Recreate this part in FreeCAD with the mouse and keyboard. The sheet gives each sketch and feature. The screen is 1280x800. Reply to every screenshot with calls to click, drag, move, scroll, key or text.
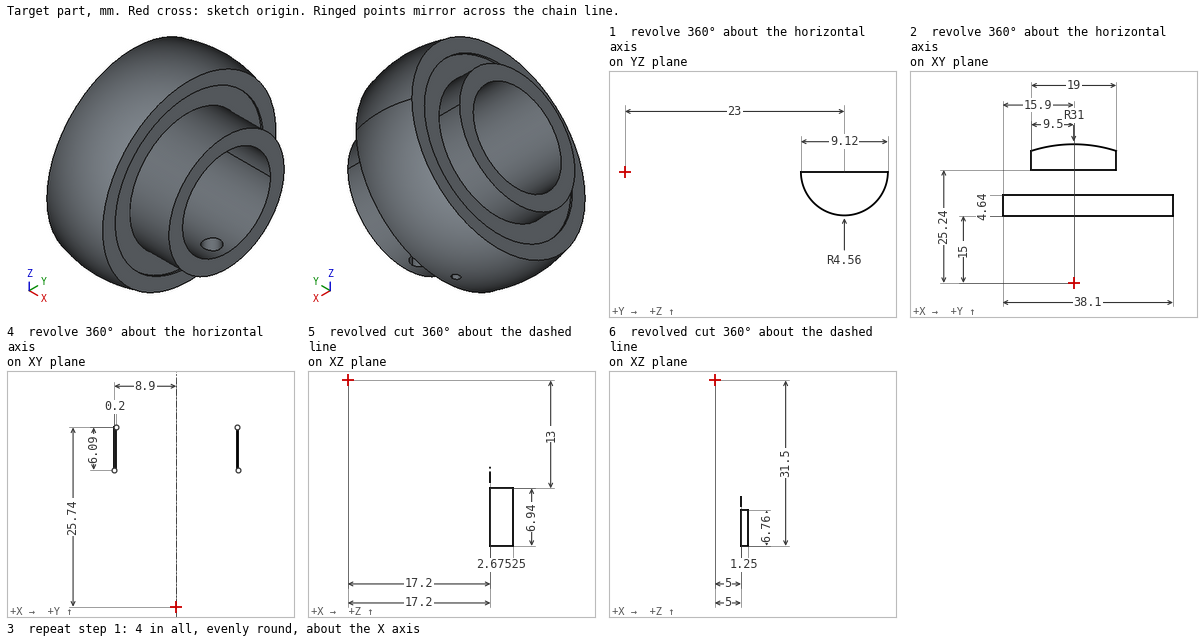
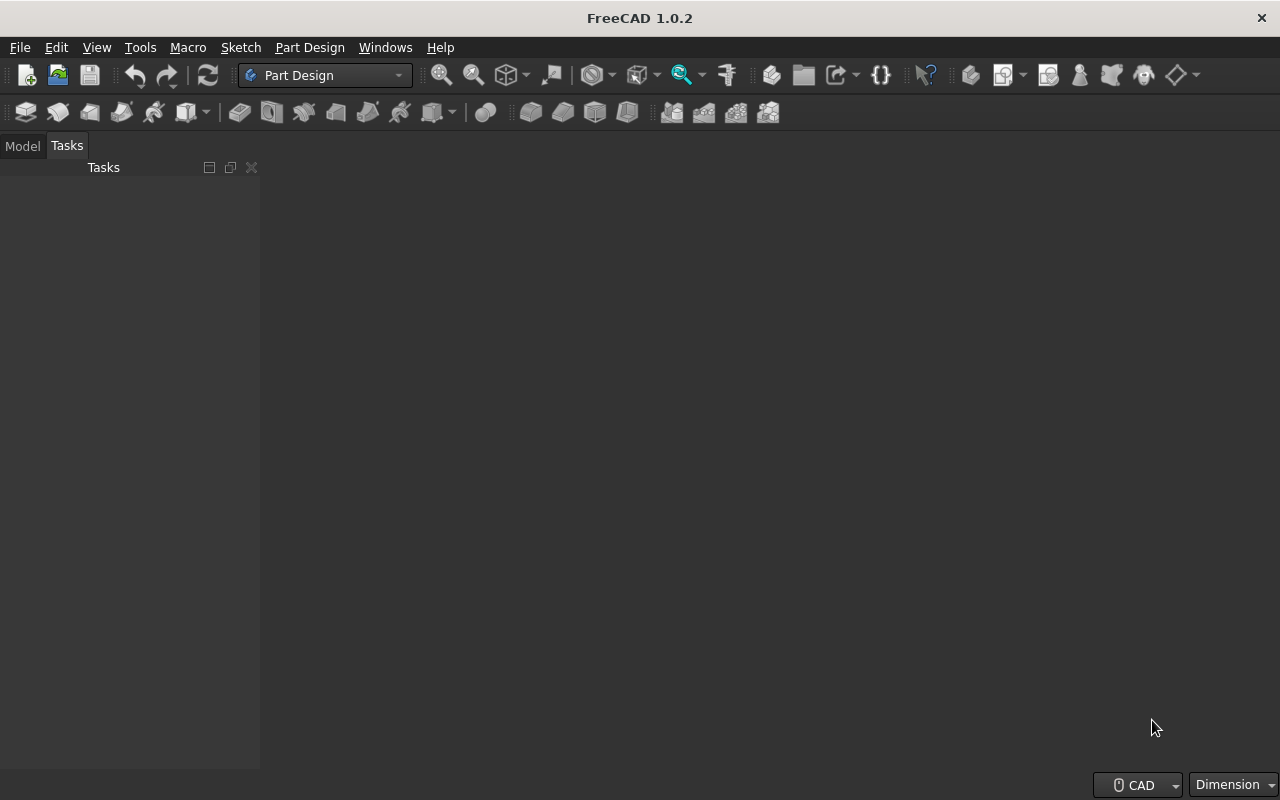
click(26, 76)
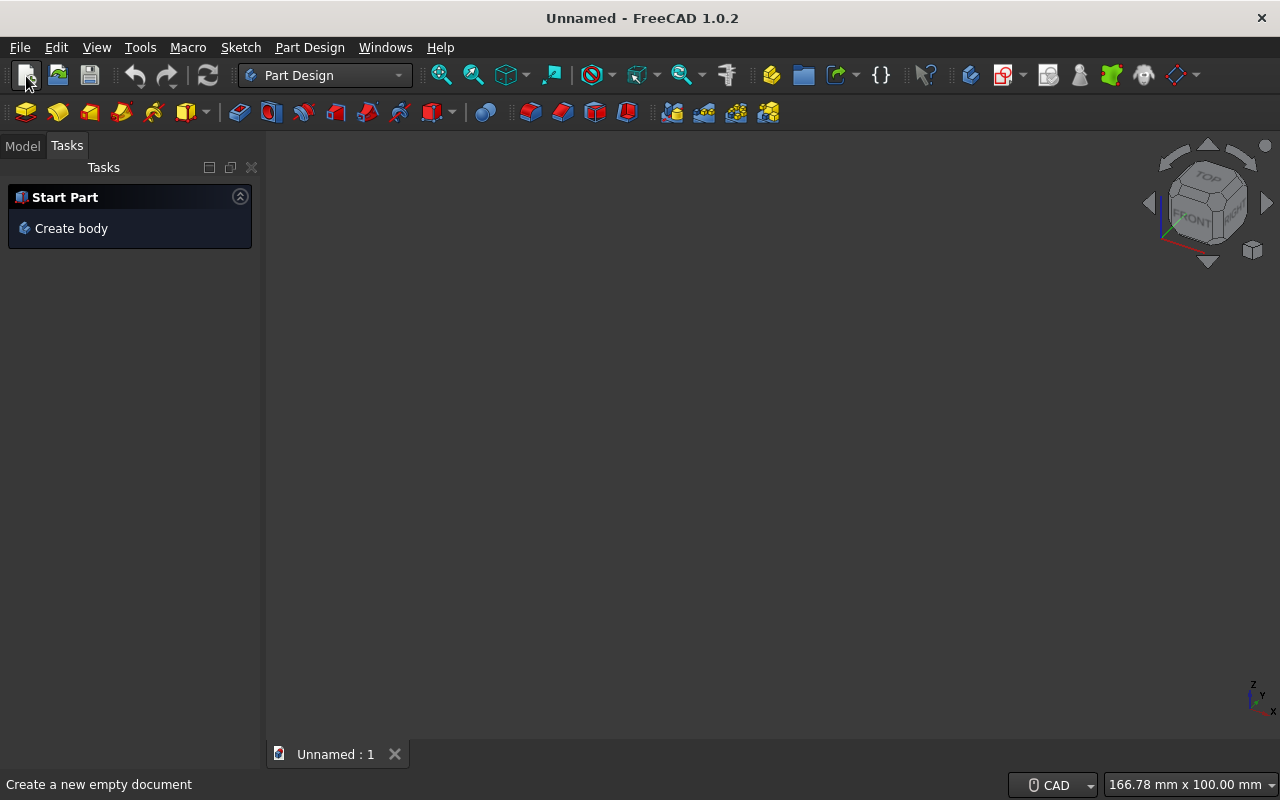
click(1004, 76)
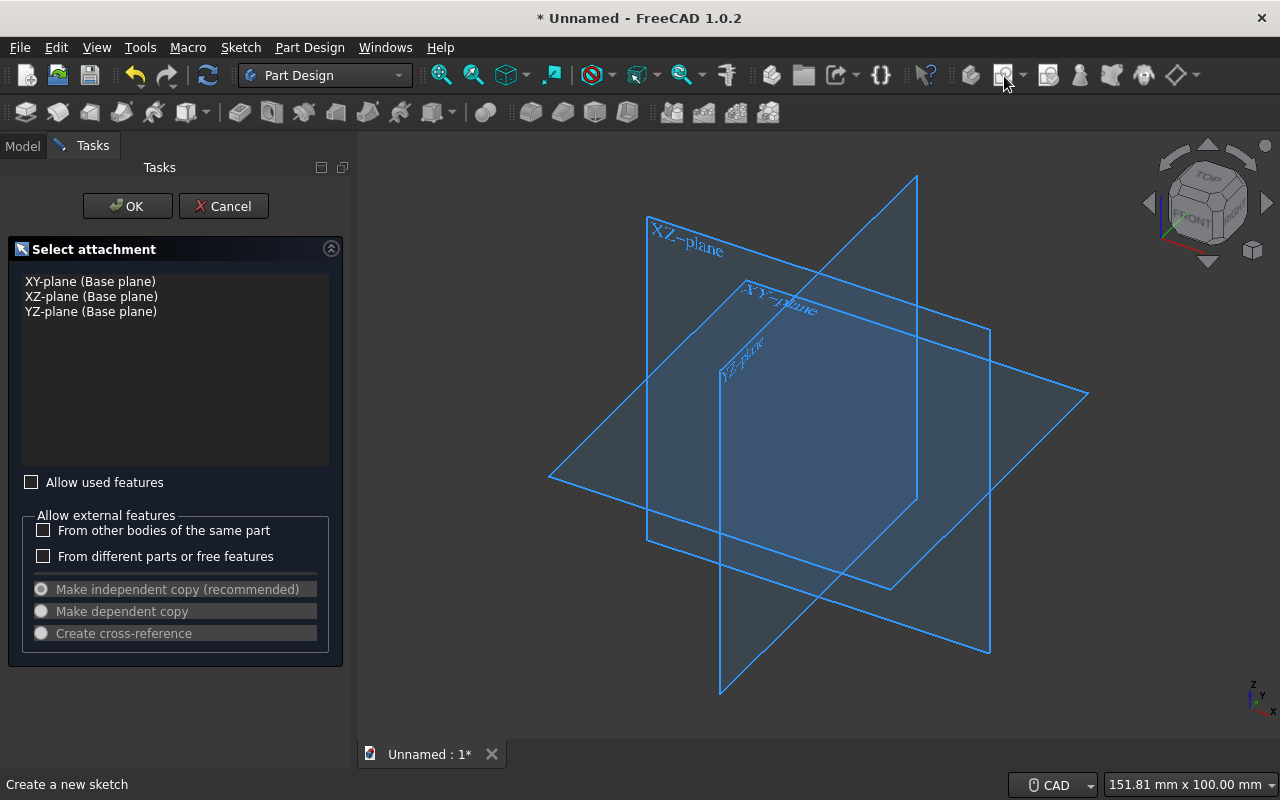
click(82, 312)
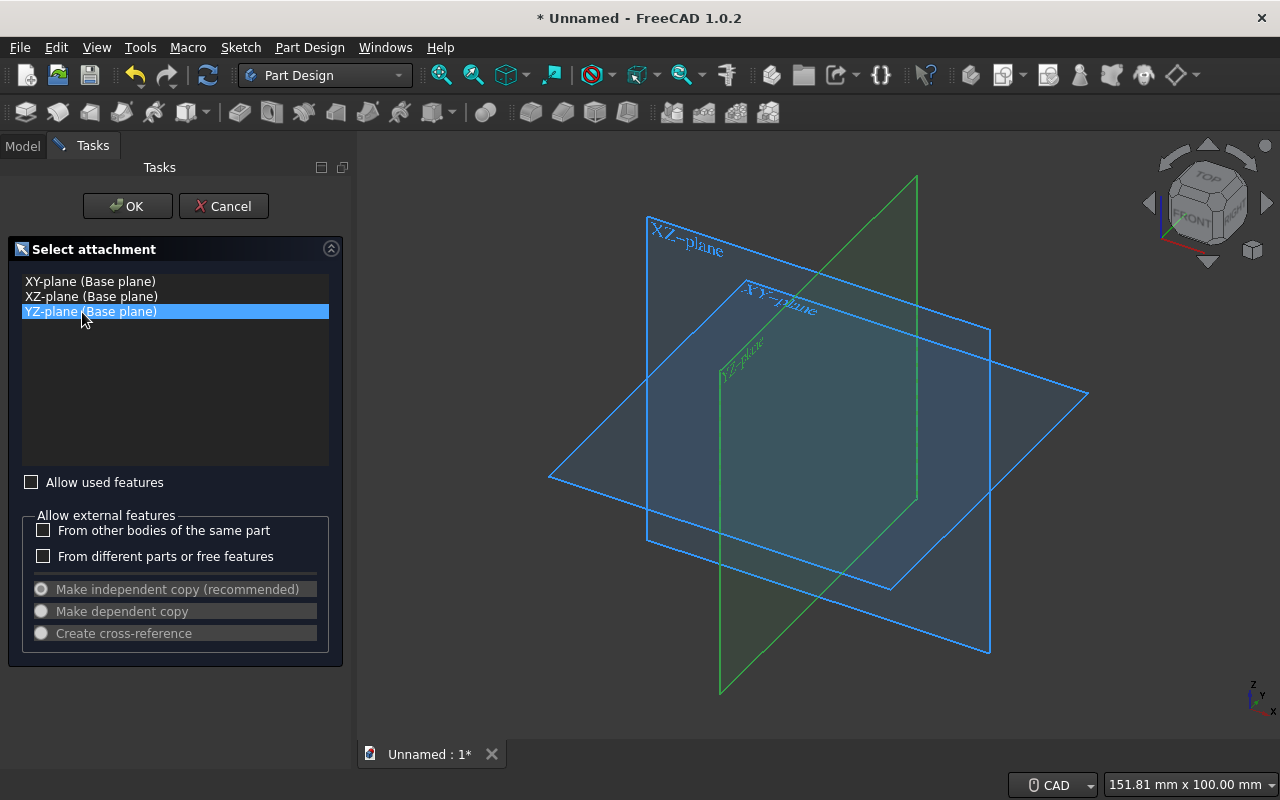
click(128, 206)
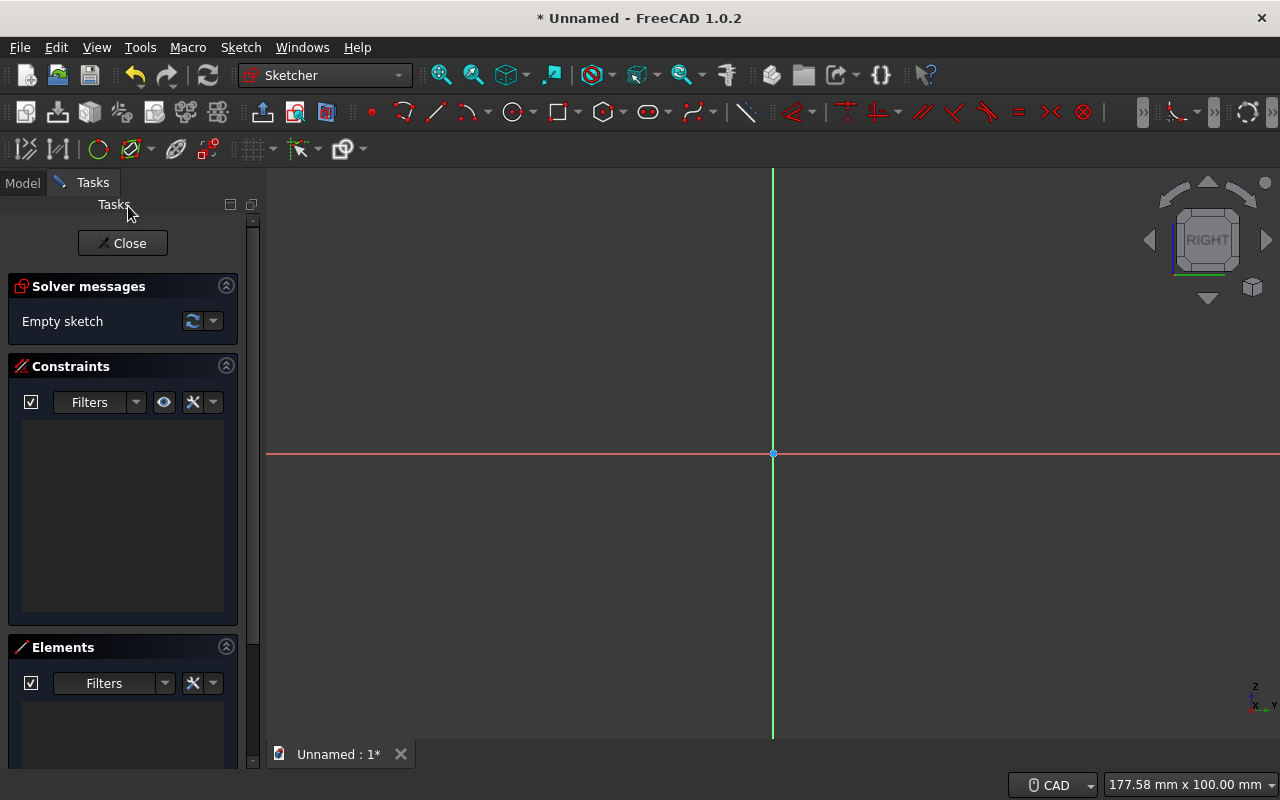
scroll(924, 468, up, 12)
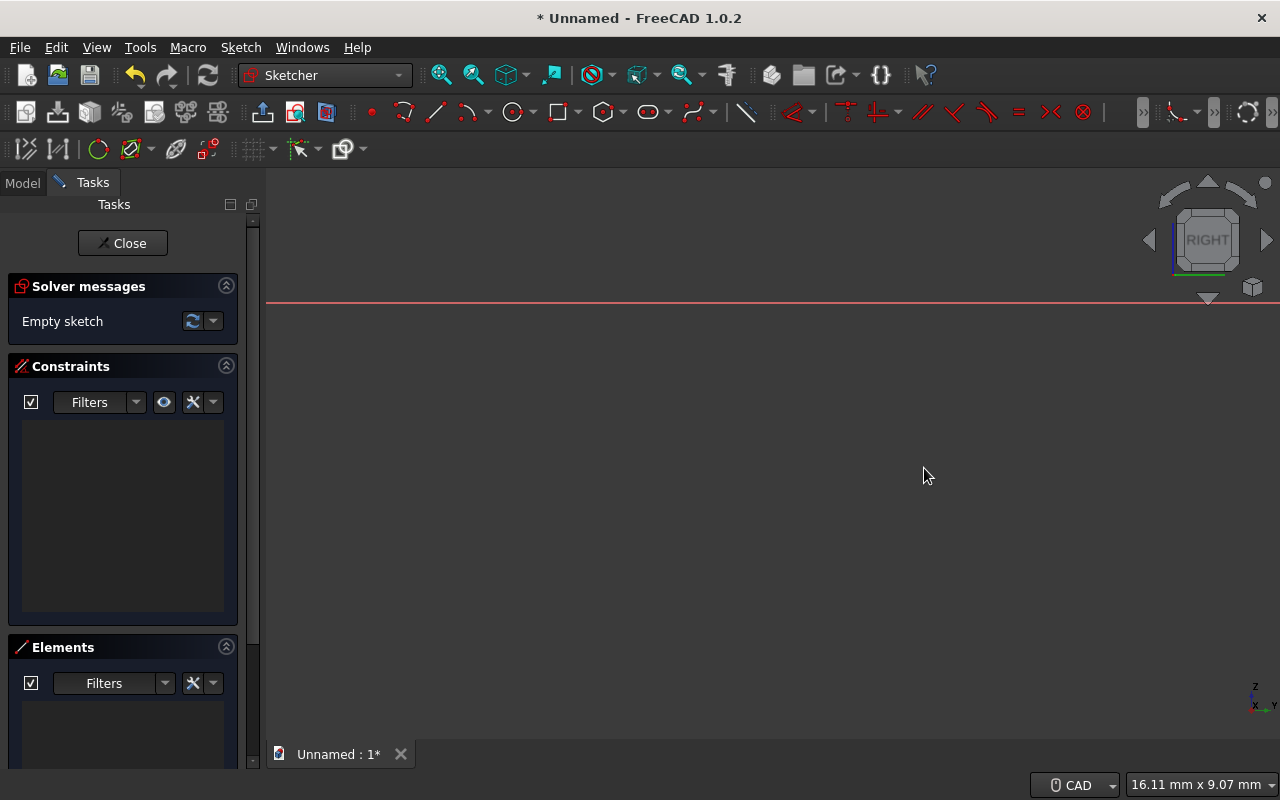
click(436, 112)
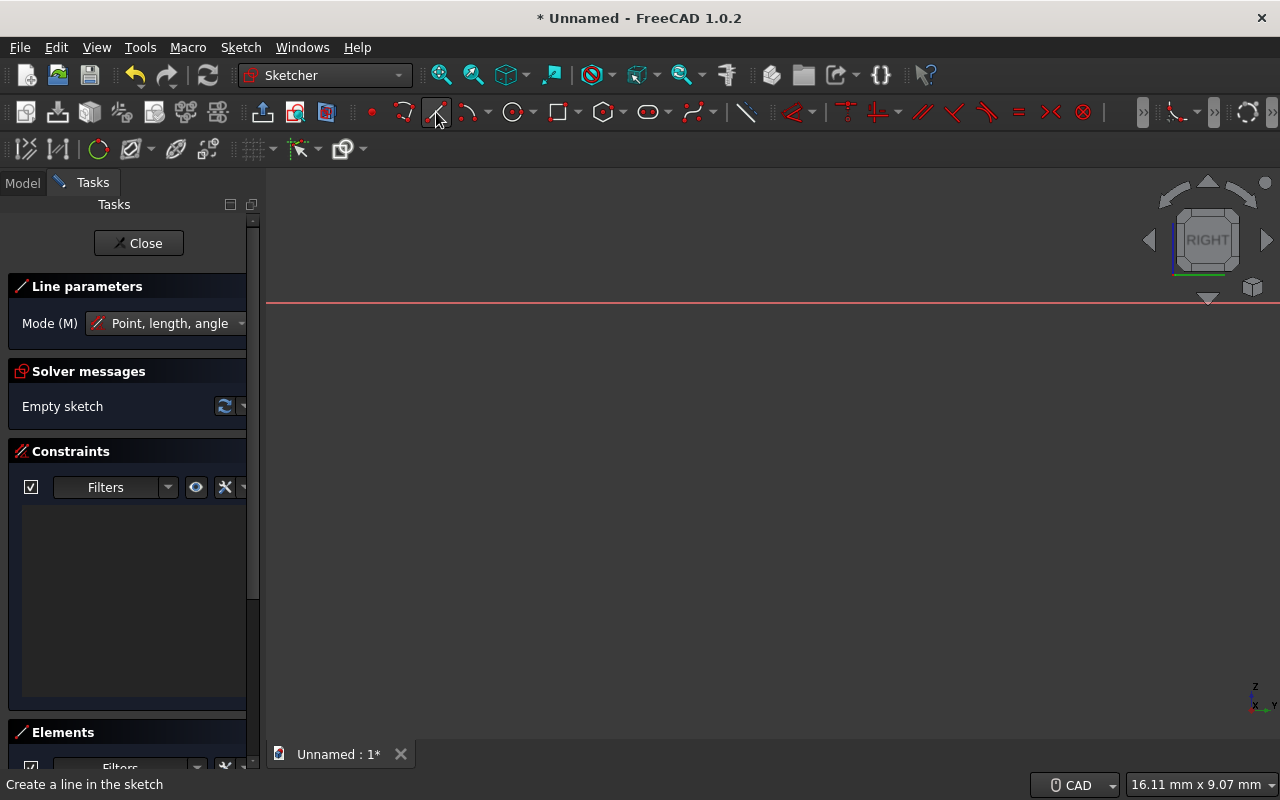
click(988, 303)
click(414, 312)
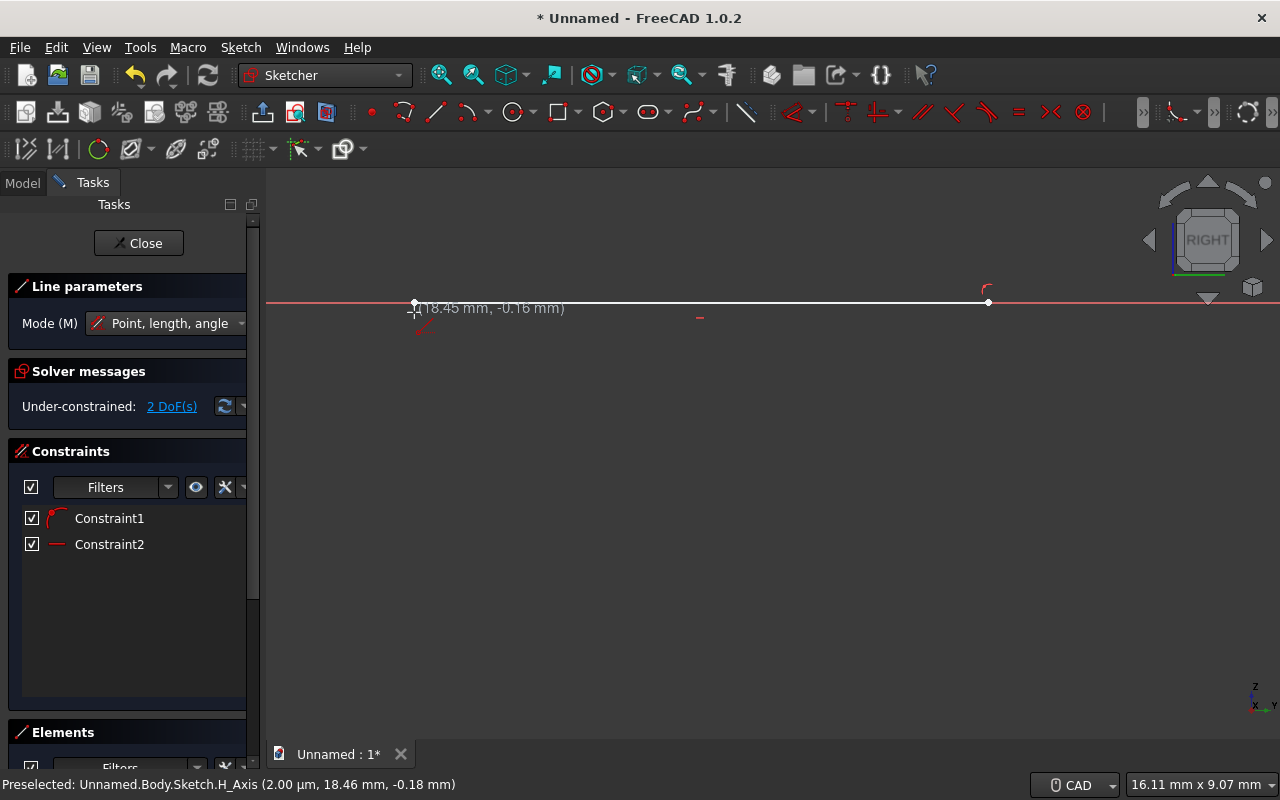
key(g)
key(3)
key(a)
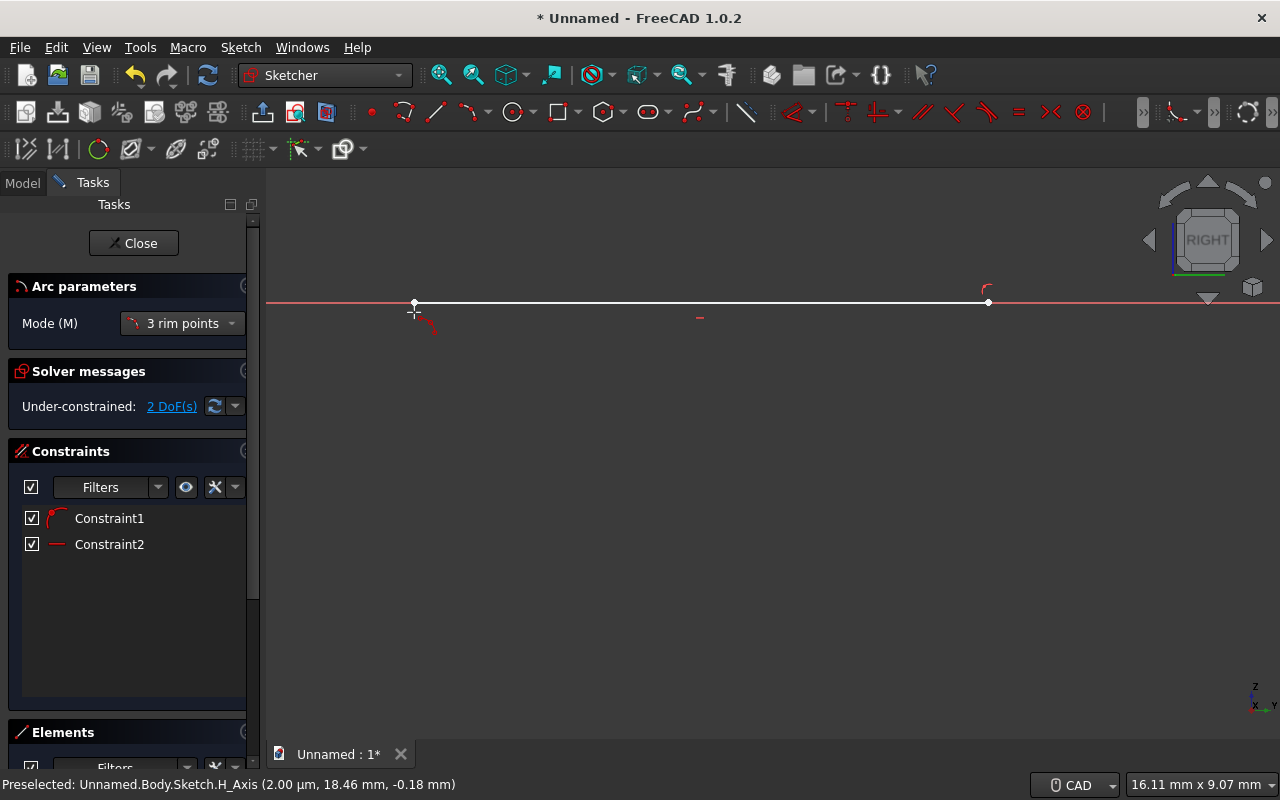
click(414, 312)
click(988, 303)
click(701, 590)
key(Escape)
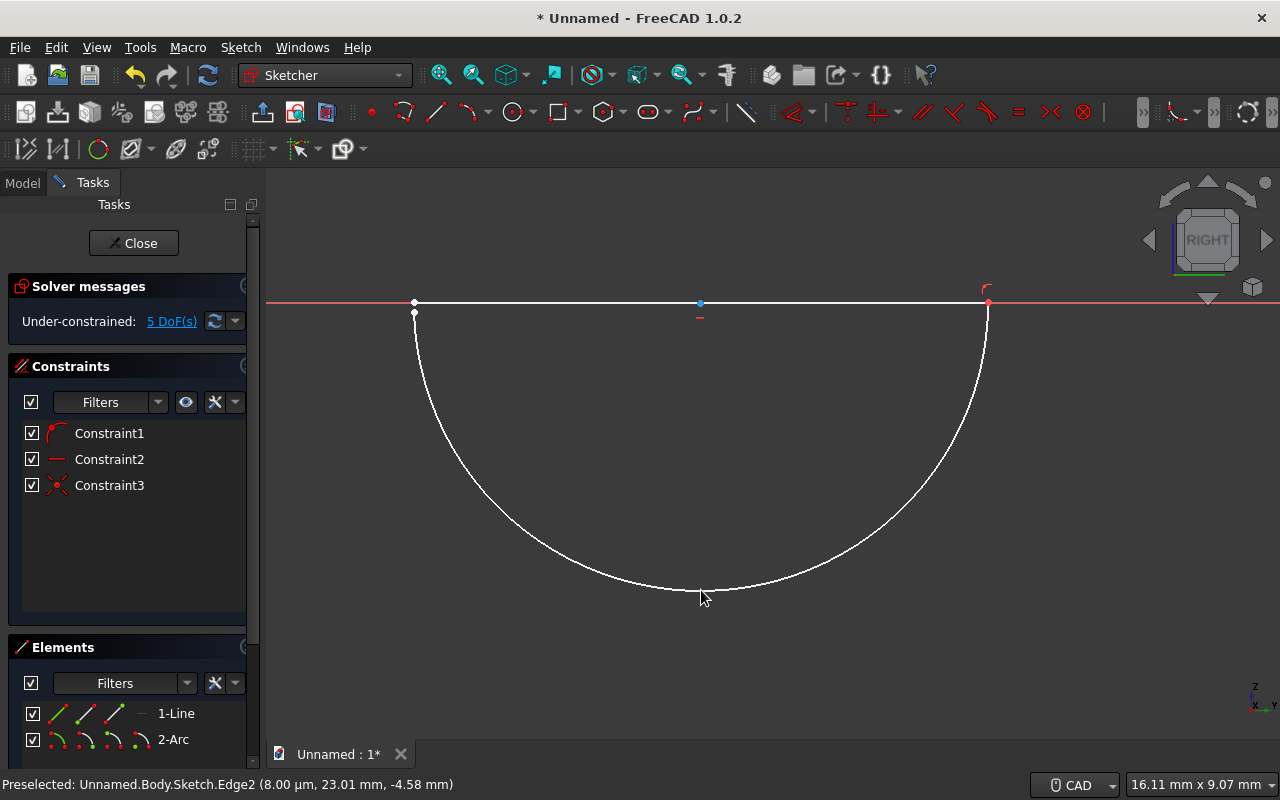
click(701, 304)